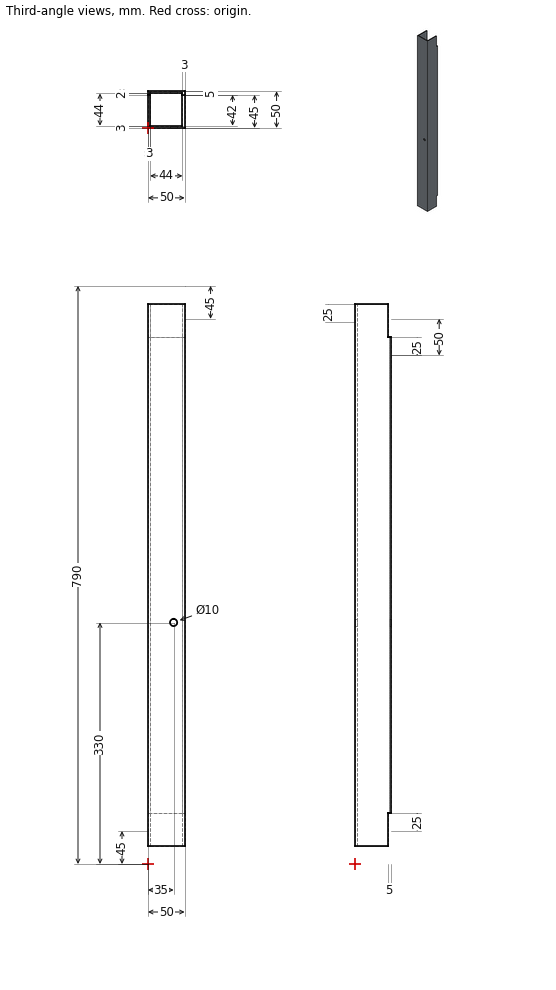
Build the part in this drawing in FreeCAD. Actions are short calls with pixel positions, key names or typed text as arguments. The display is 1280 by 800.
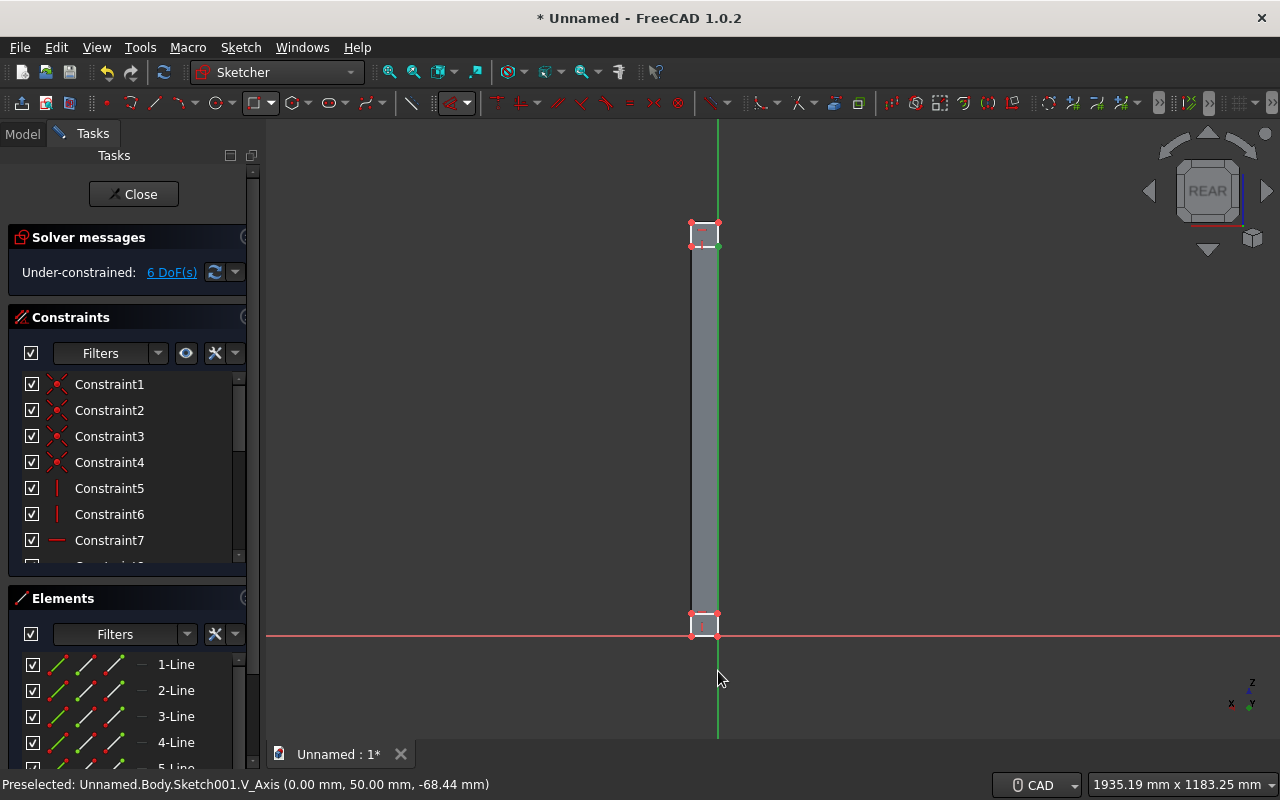
key(c)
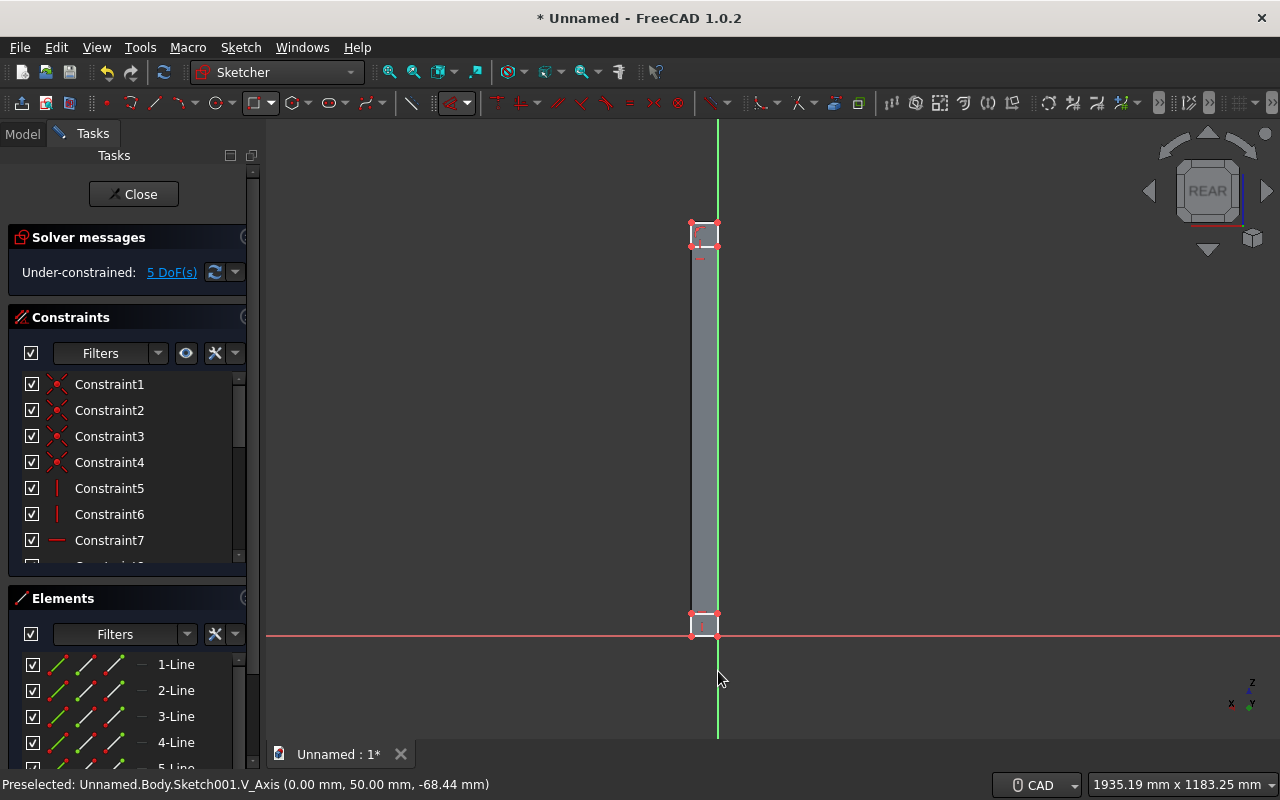
click(450, 104)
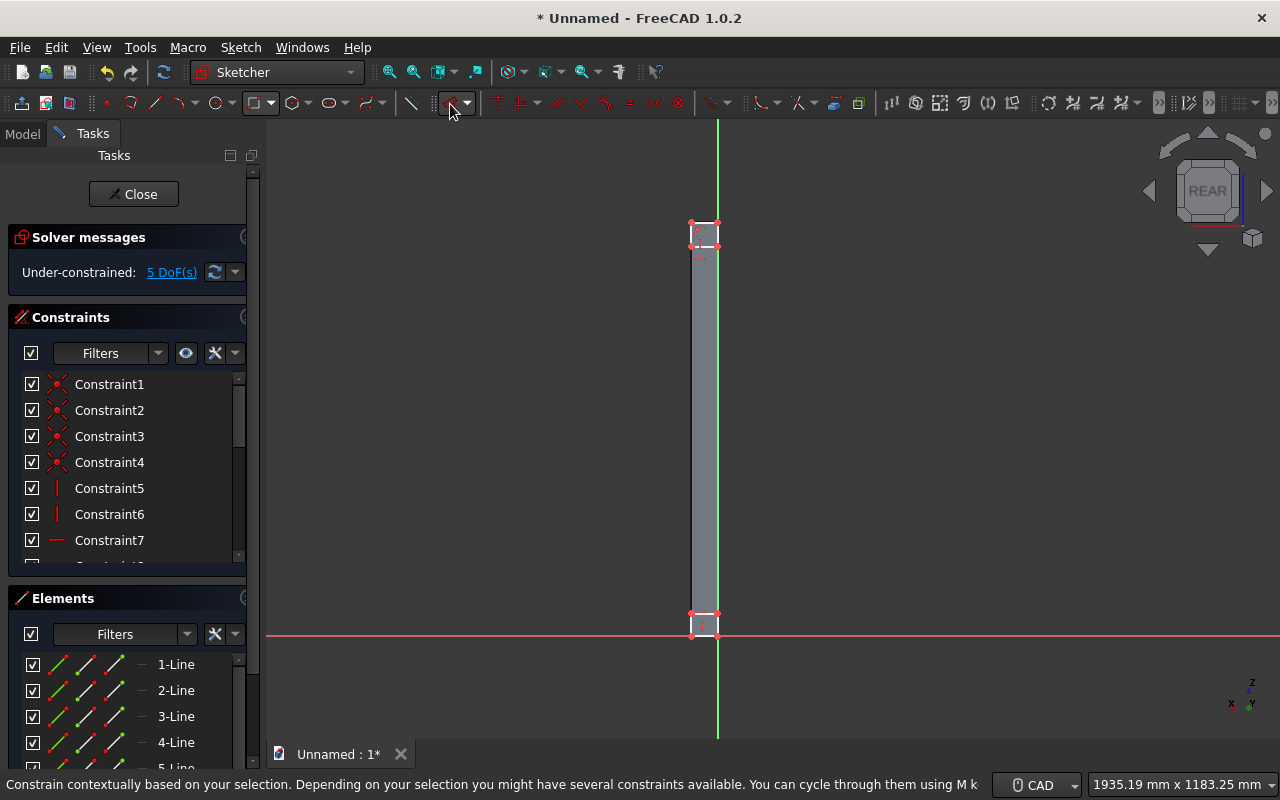
scroll(718, 625, up, 3)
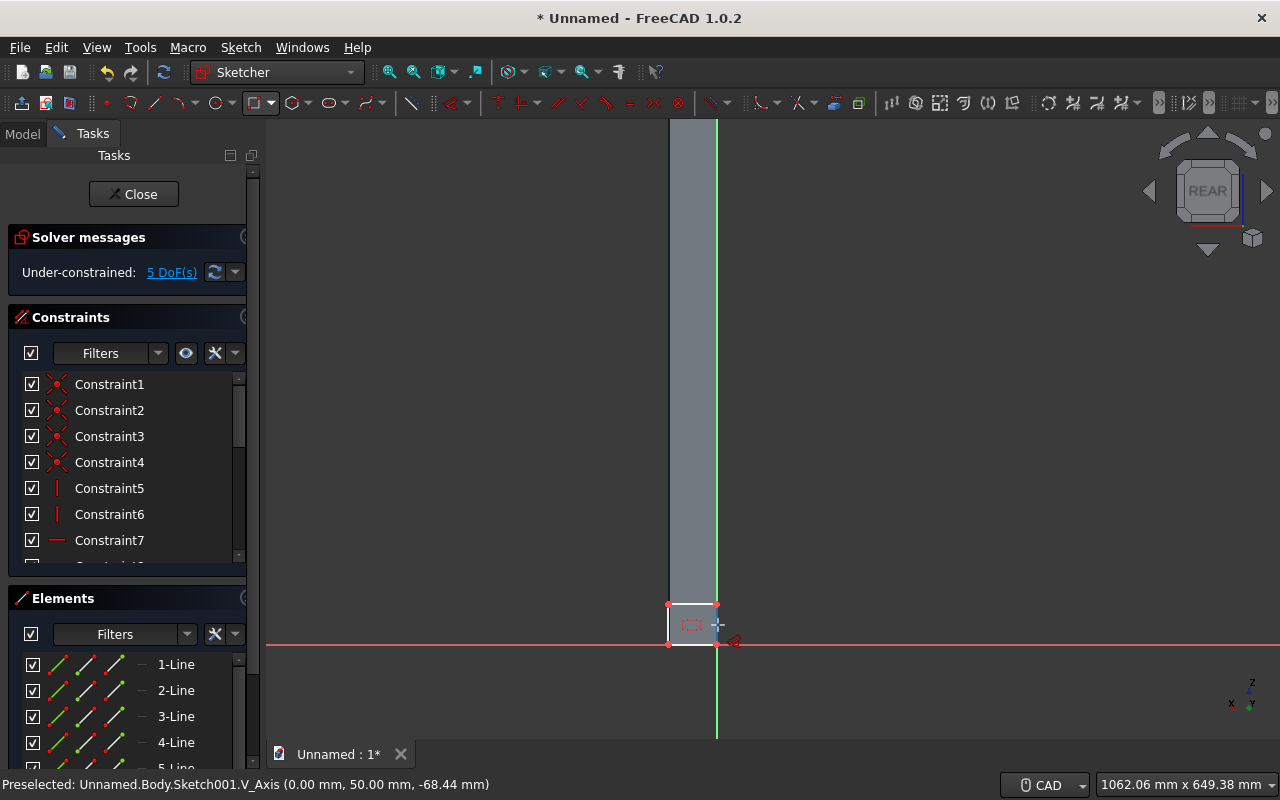
click(717, 624)
click(751, 624)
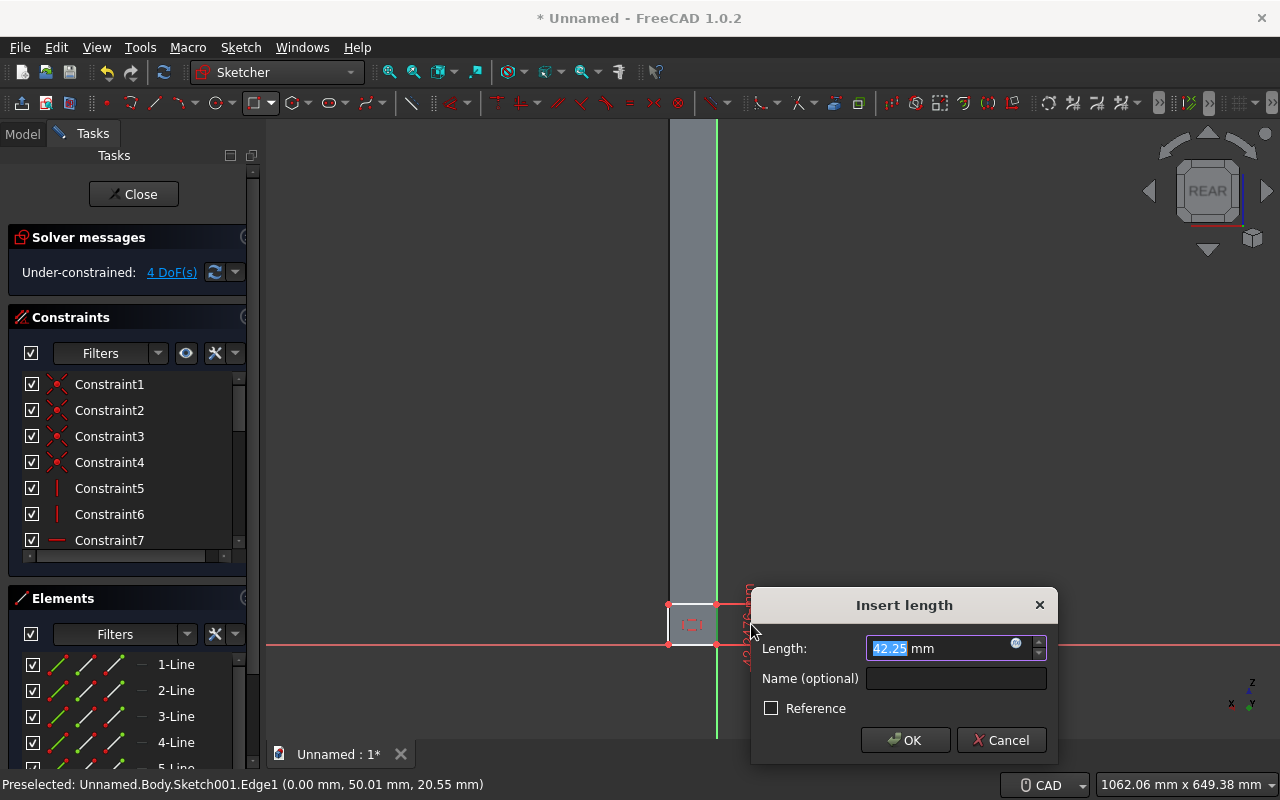
text(45)
key(Return)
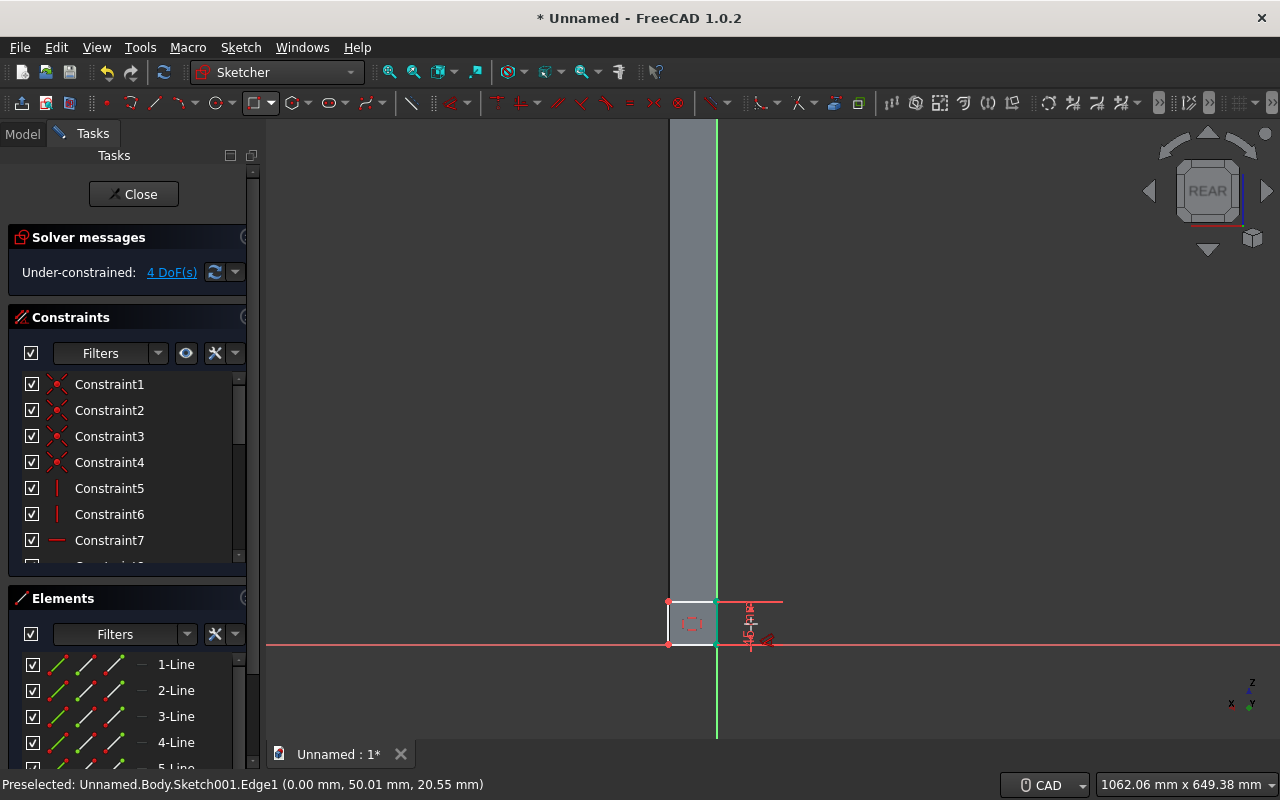
click(702, 602)
click(693, 568)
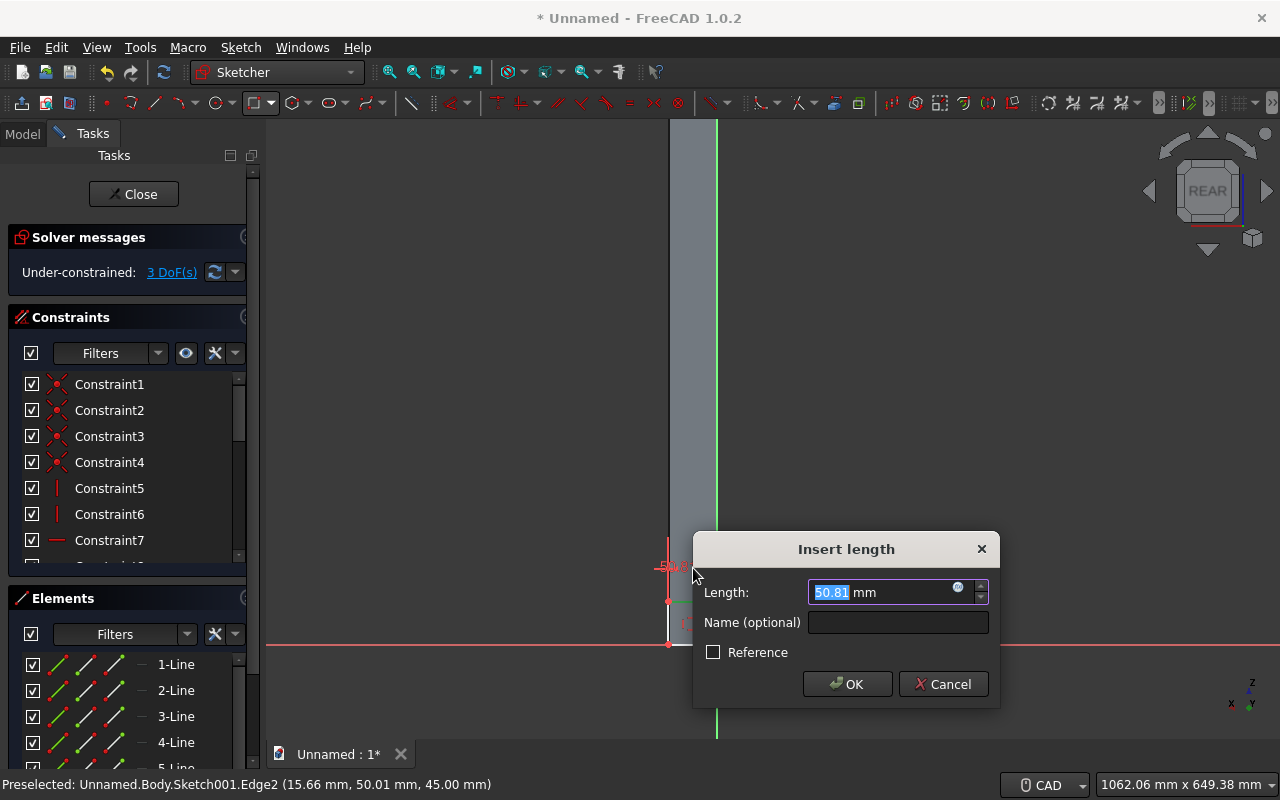
text(50)
key(Return)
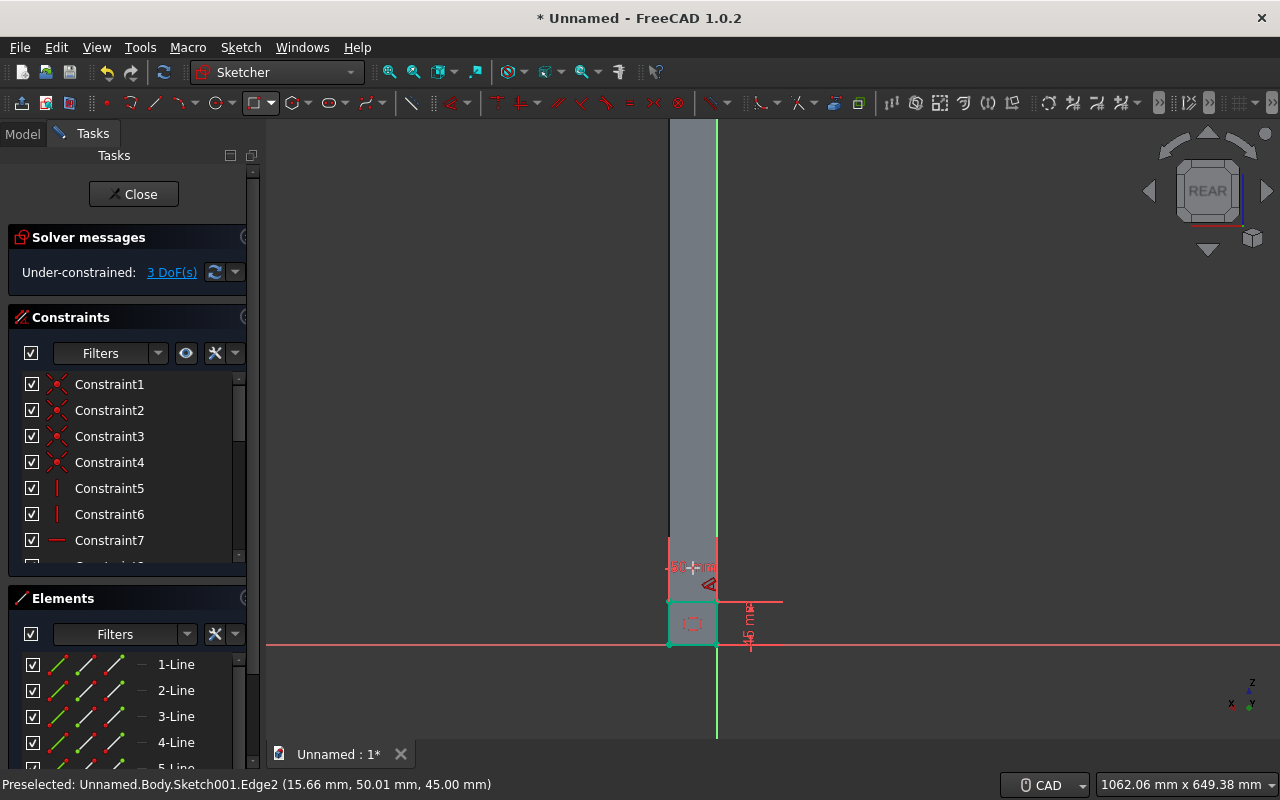
scroll(718, 625, down, 3)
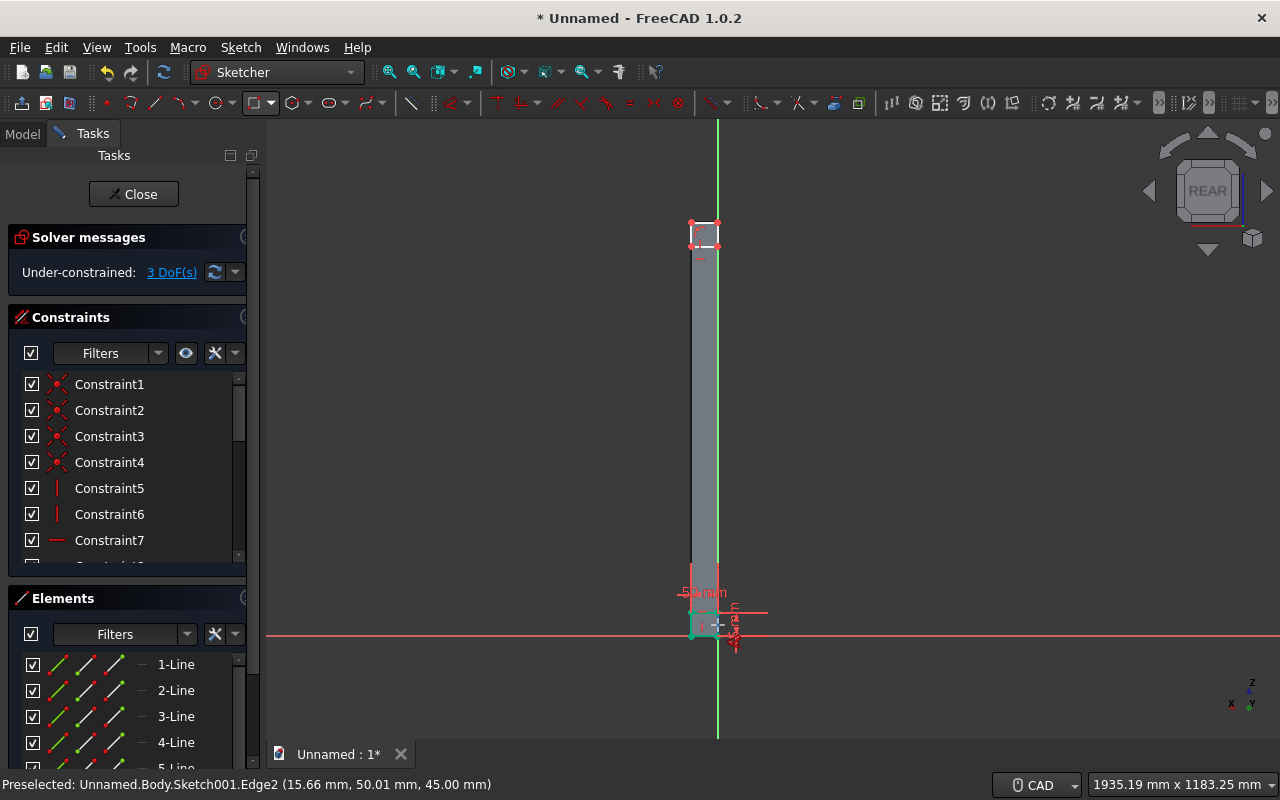
scroll(691, 230, up, 4)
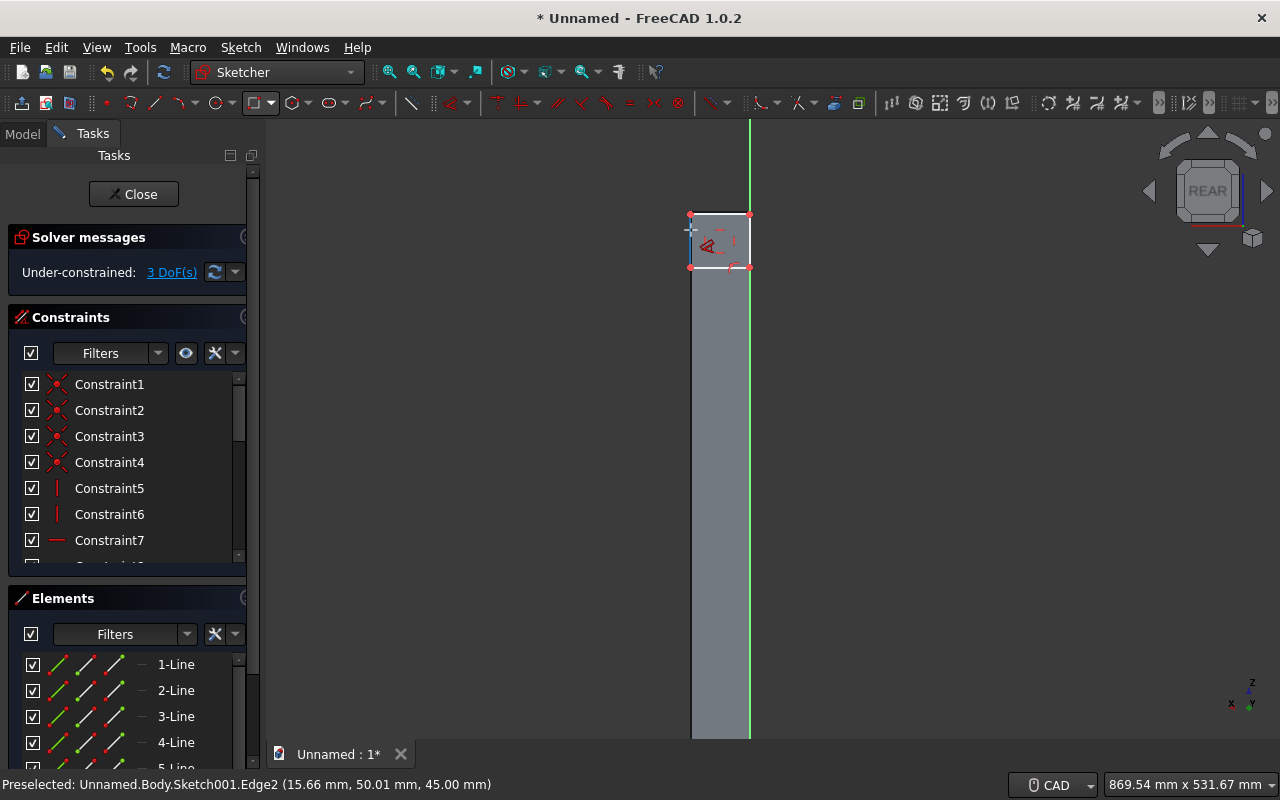
click(690, 230)
click(656, 241)